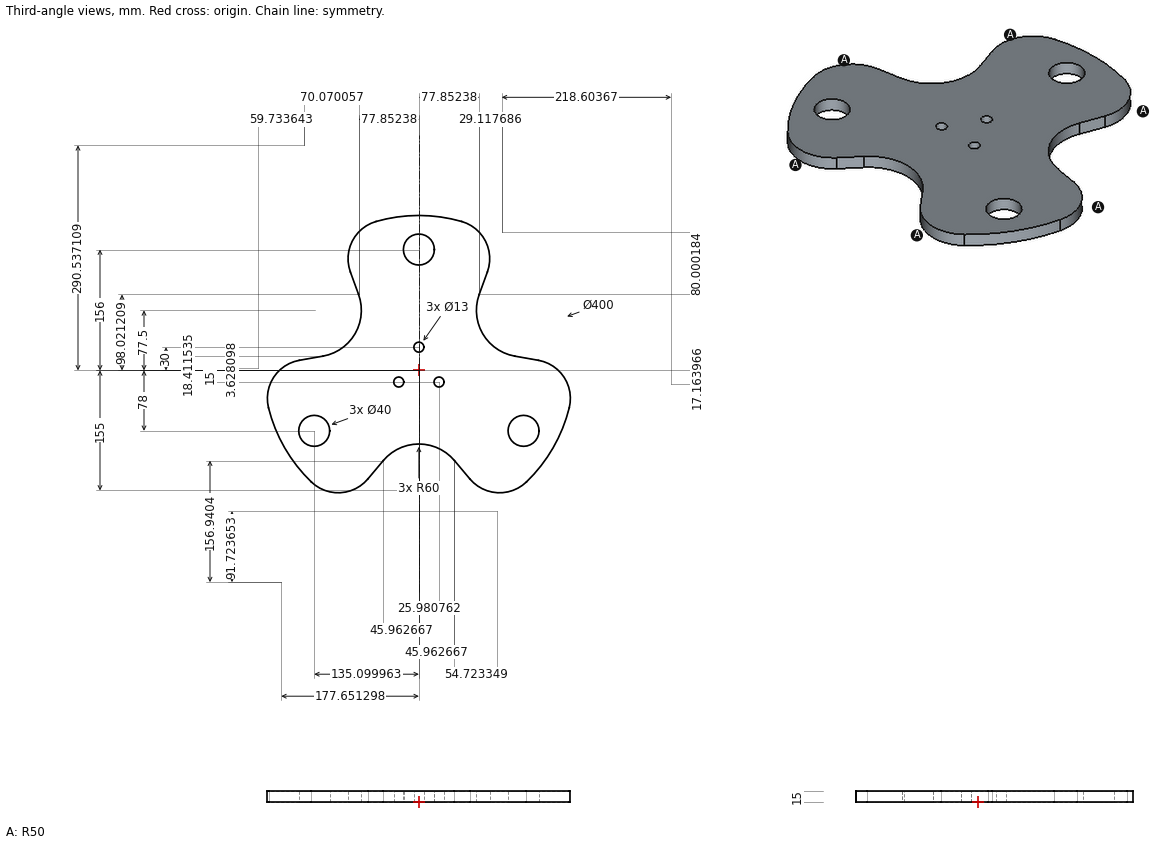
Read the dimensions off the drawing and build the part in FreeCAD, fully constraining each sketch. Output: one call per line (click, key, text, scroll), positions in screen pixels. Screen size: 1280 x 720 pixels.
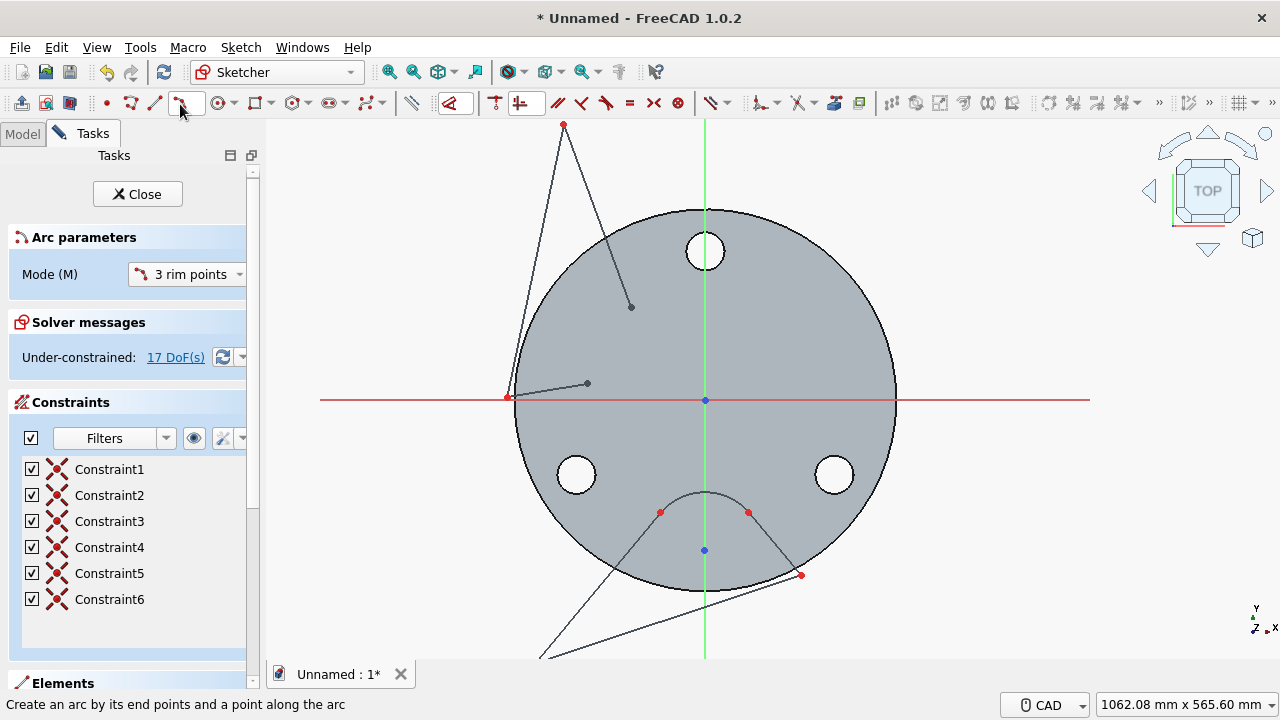
click(587, 384)
click(631, 308)
click(627, 355)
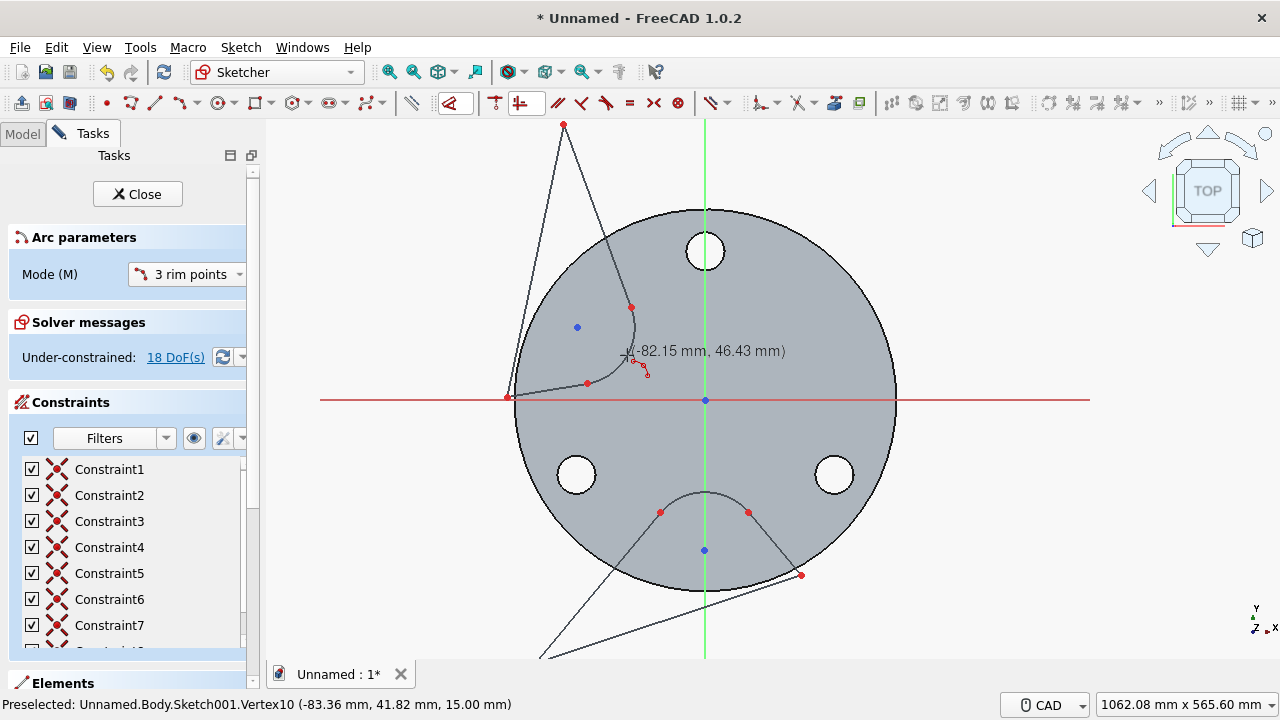
click(132, 104)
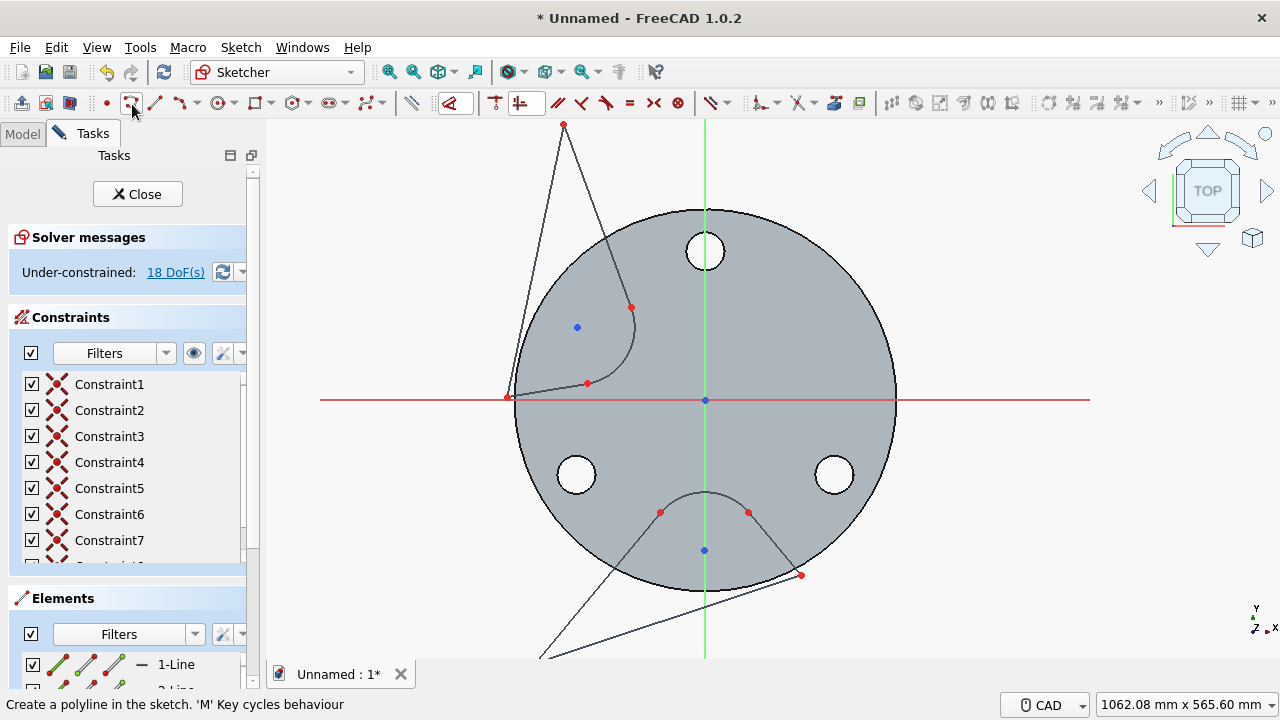
click(824, 383)
click(1016, 417)
click(808, 230)
click(780, 307)
right_click(780, 307)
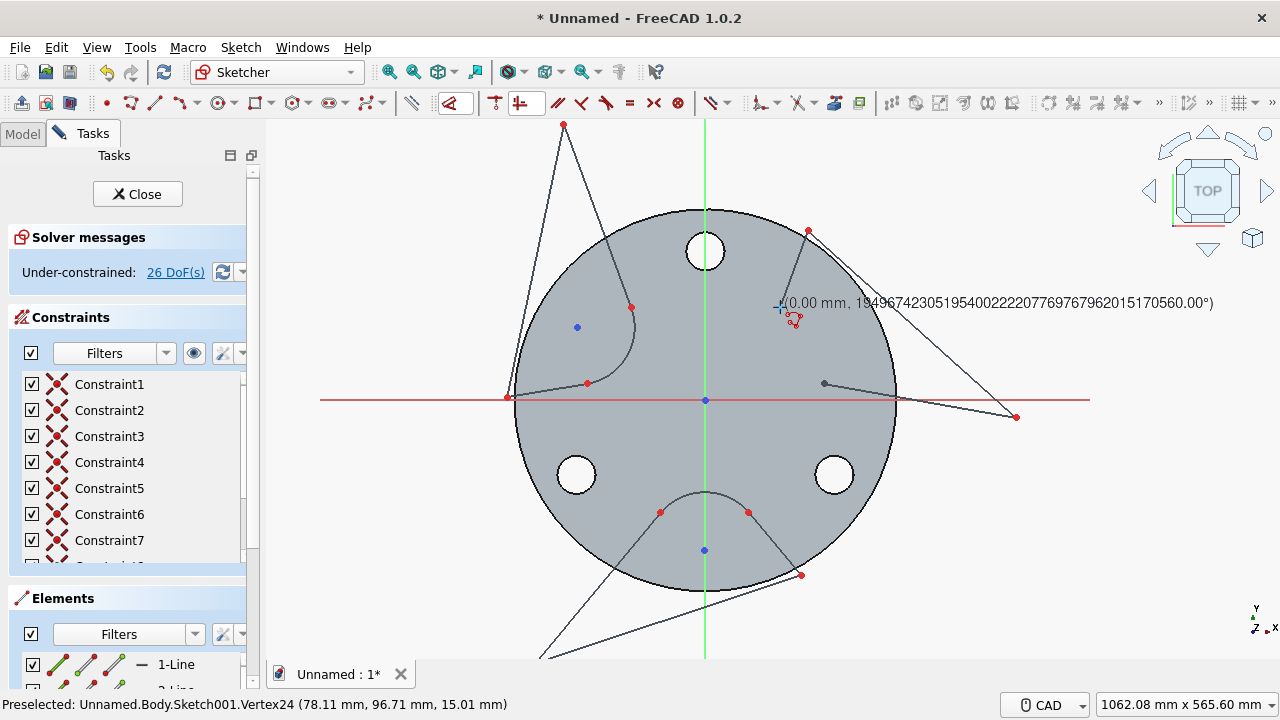
click(180, 104)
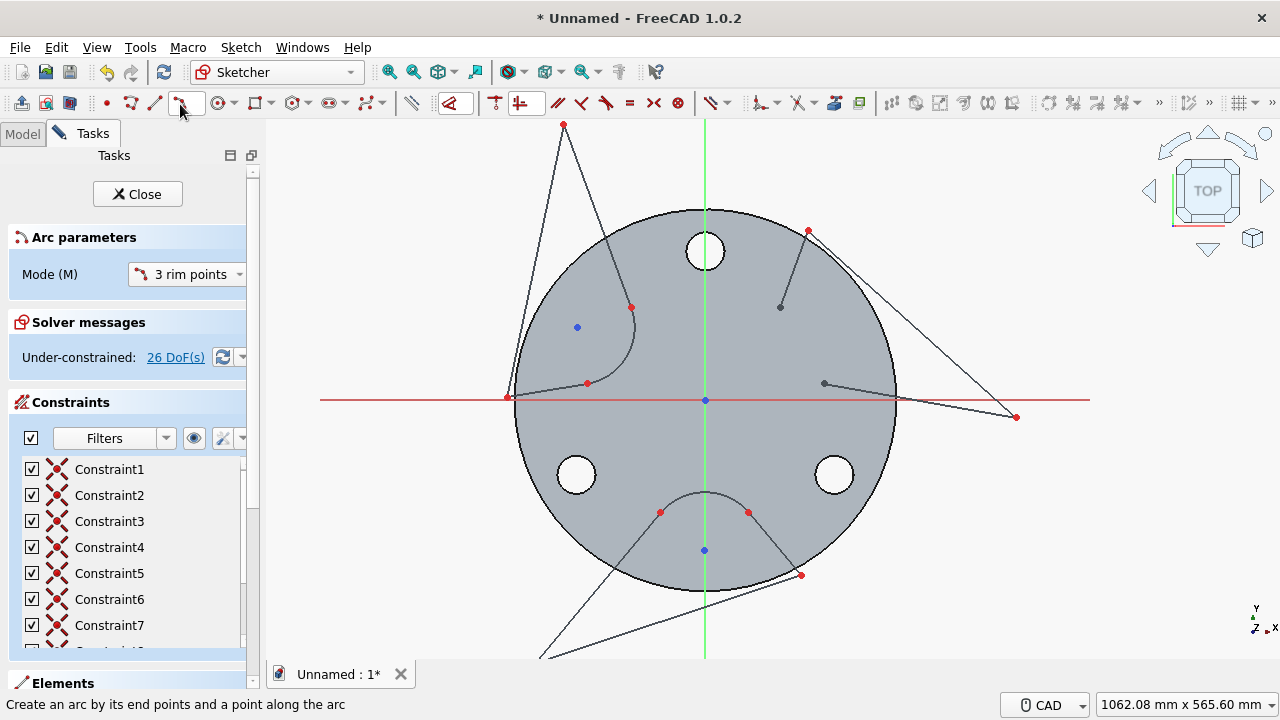
click(780, 308)
click(824, 384)
click(784, 355)
key(Escape)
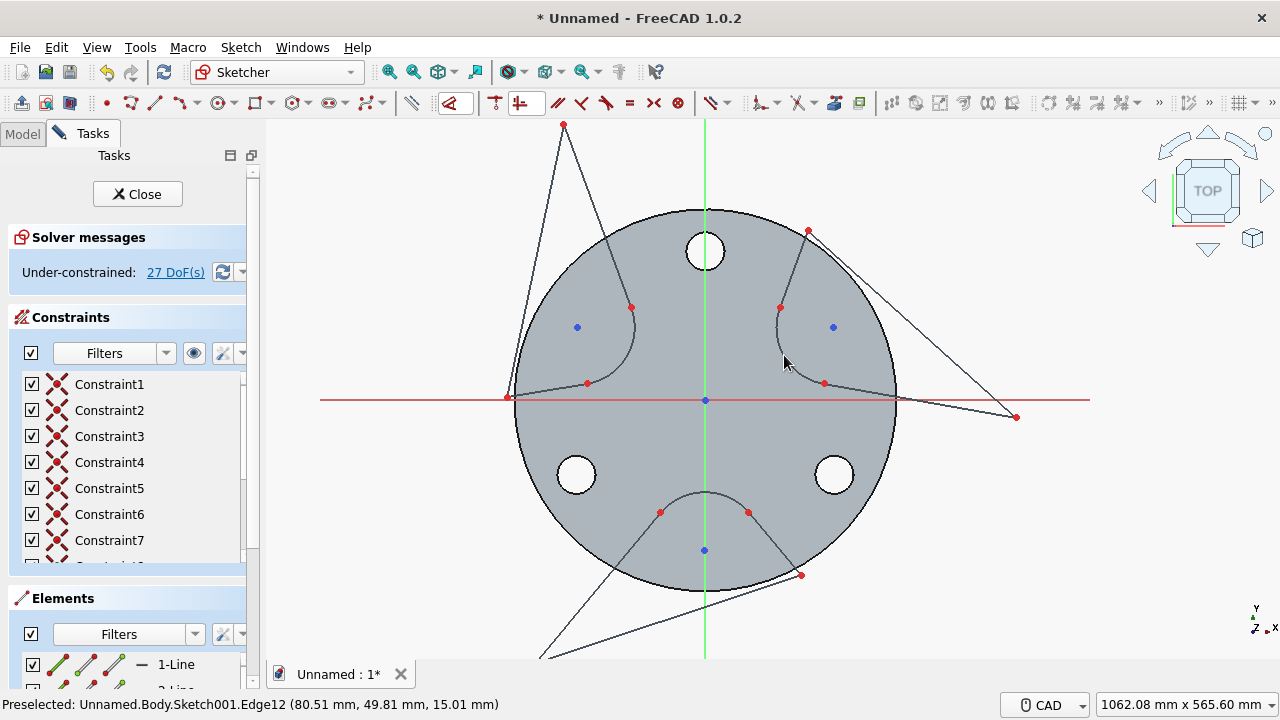
click(725, 496)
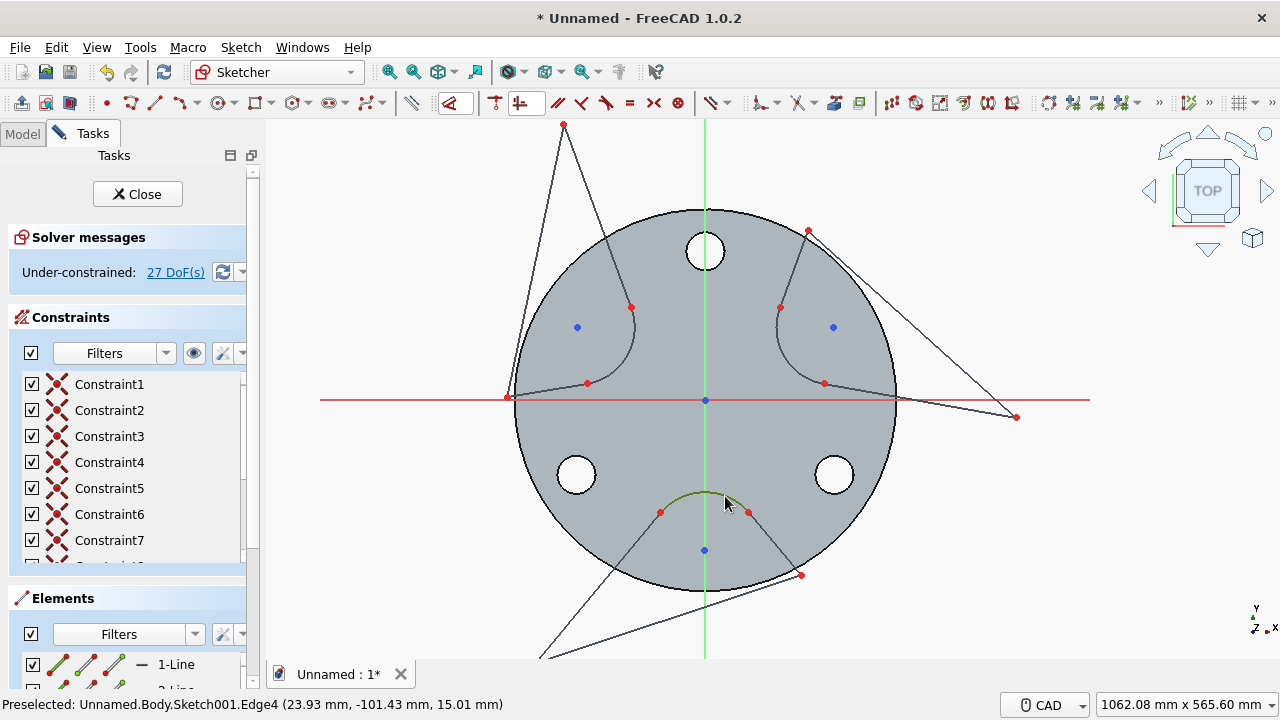
click(614, 372)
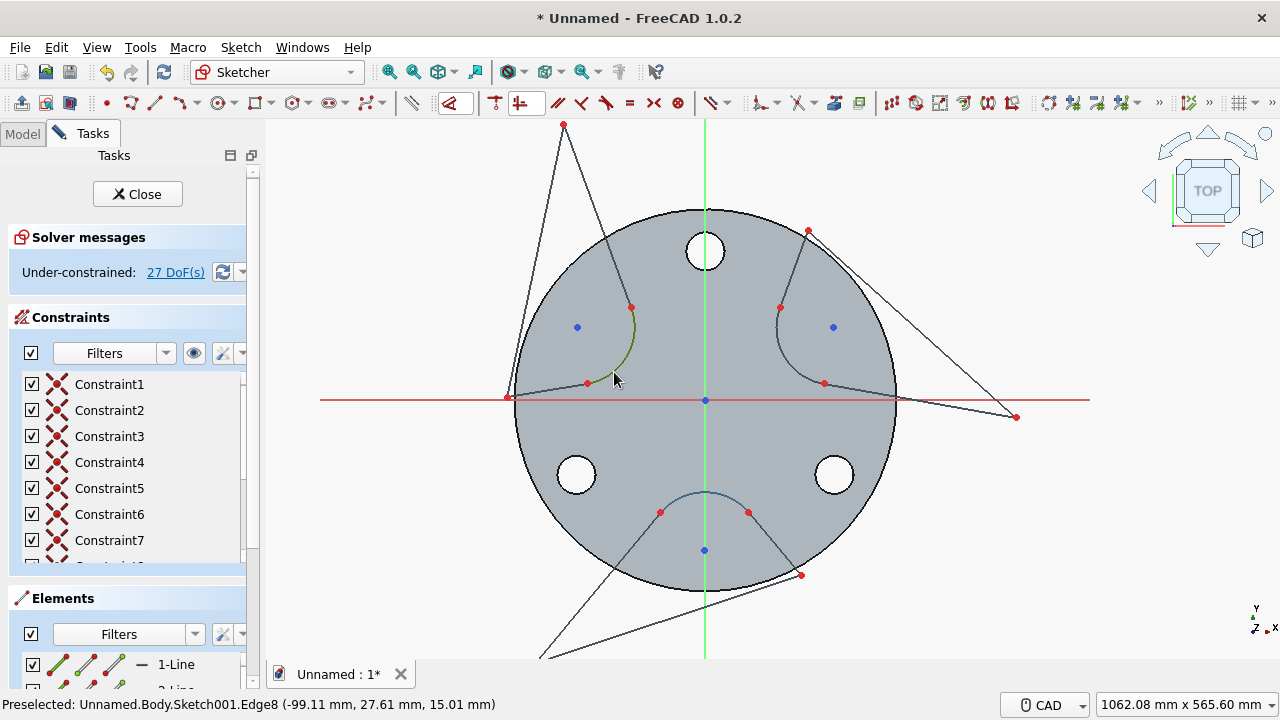
click(777, 338)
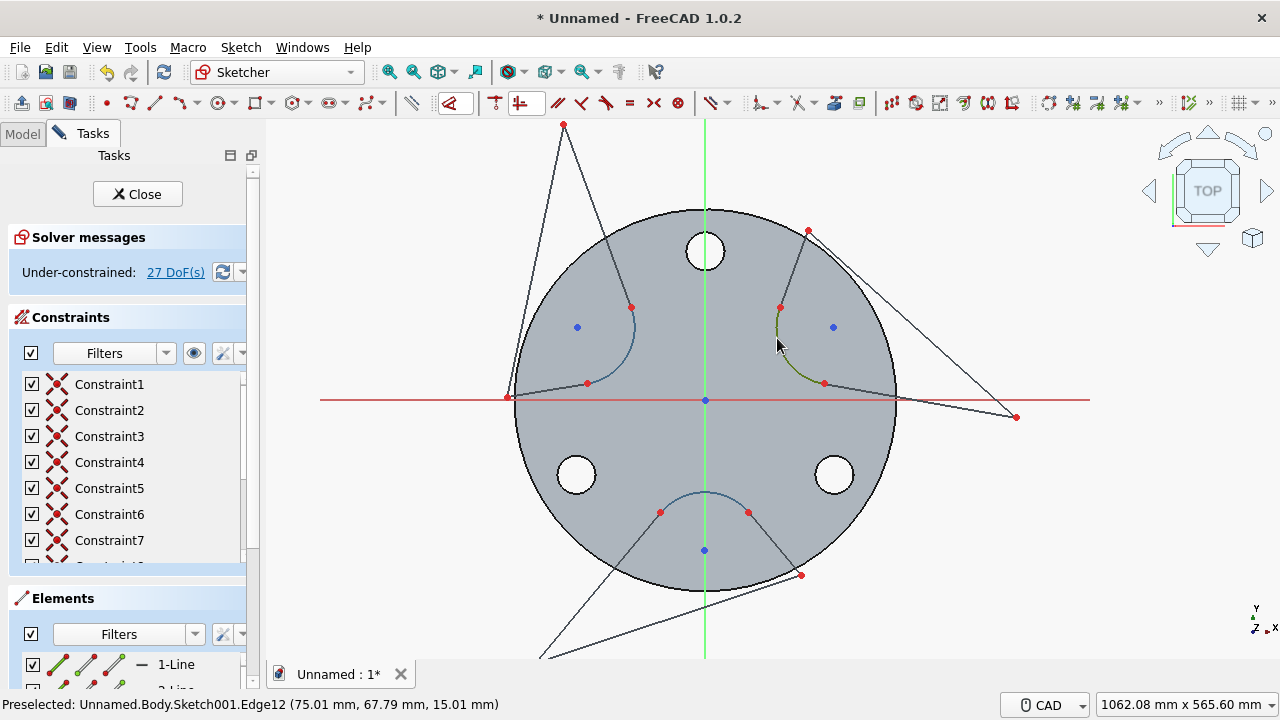
click(630, 104)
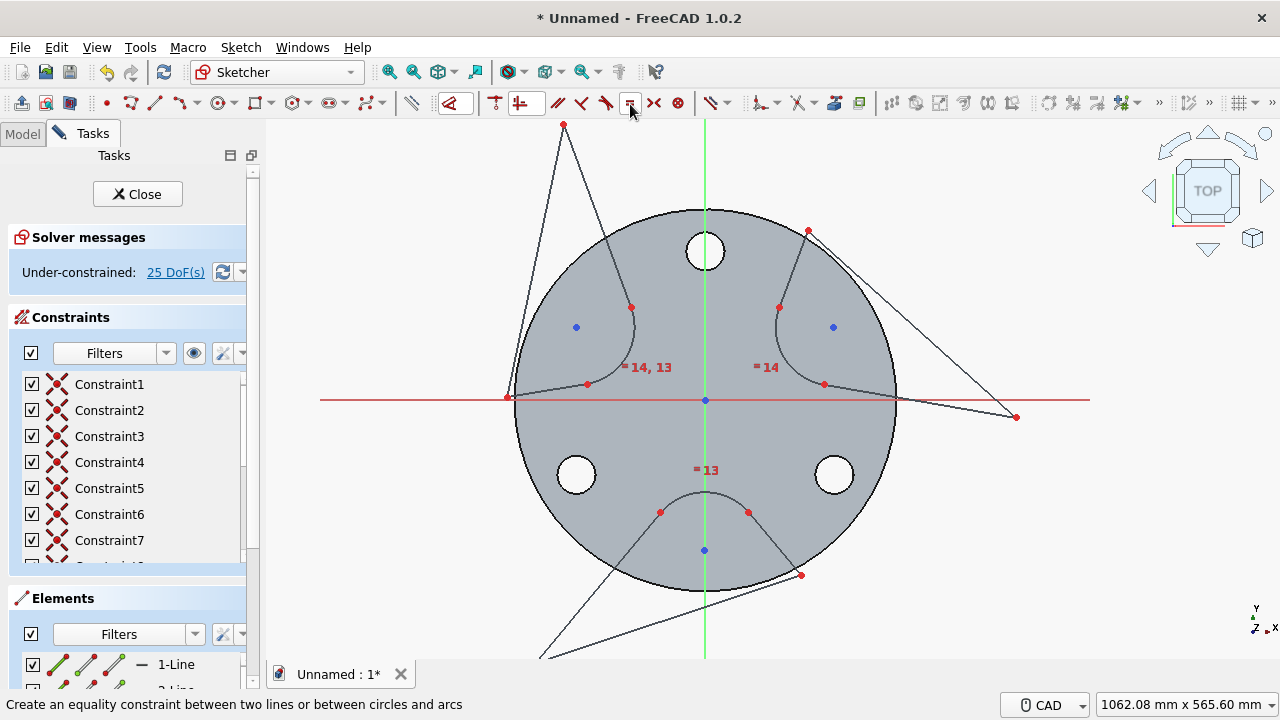
click(705, 550)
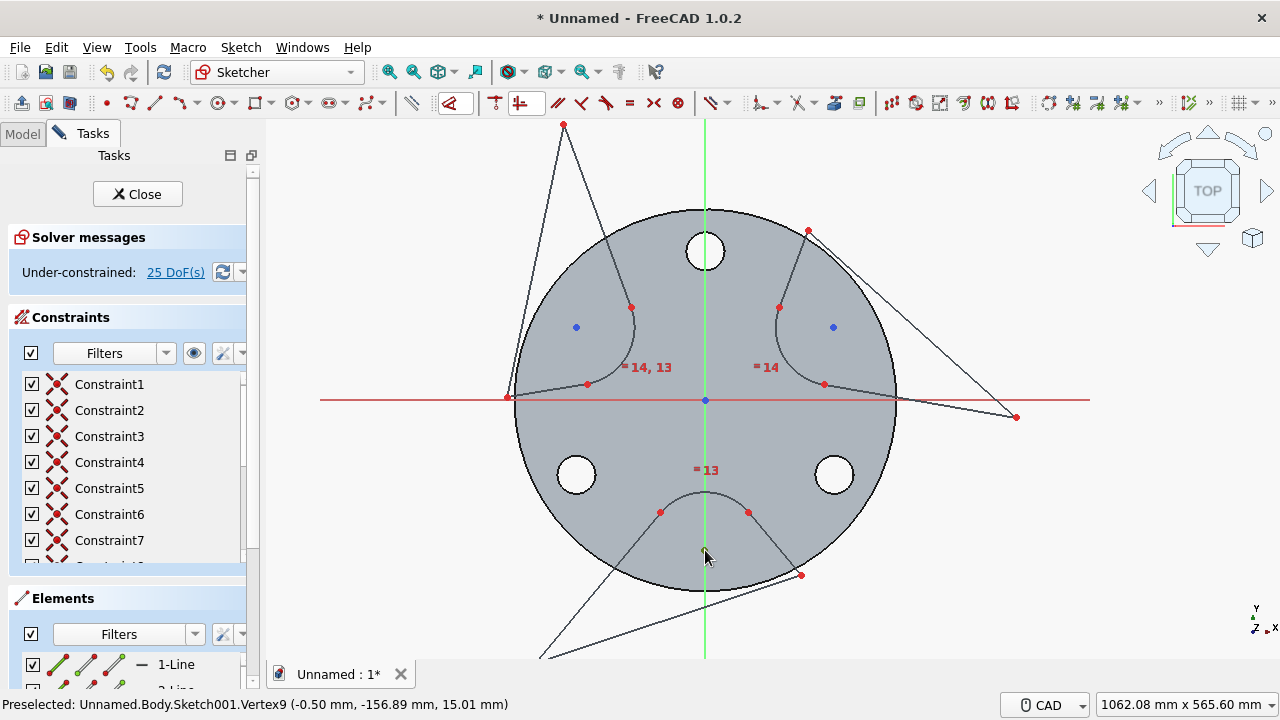
click(705, 562)